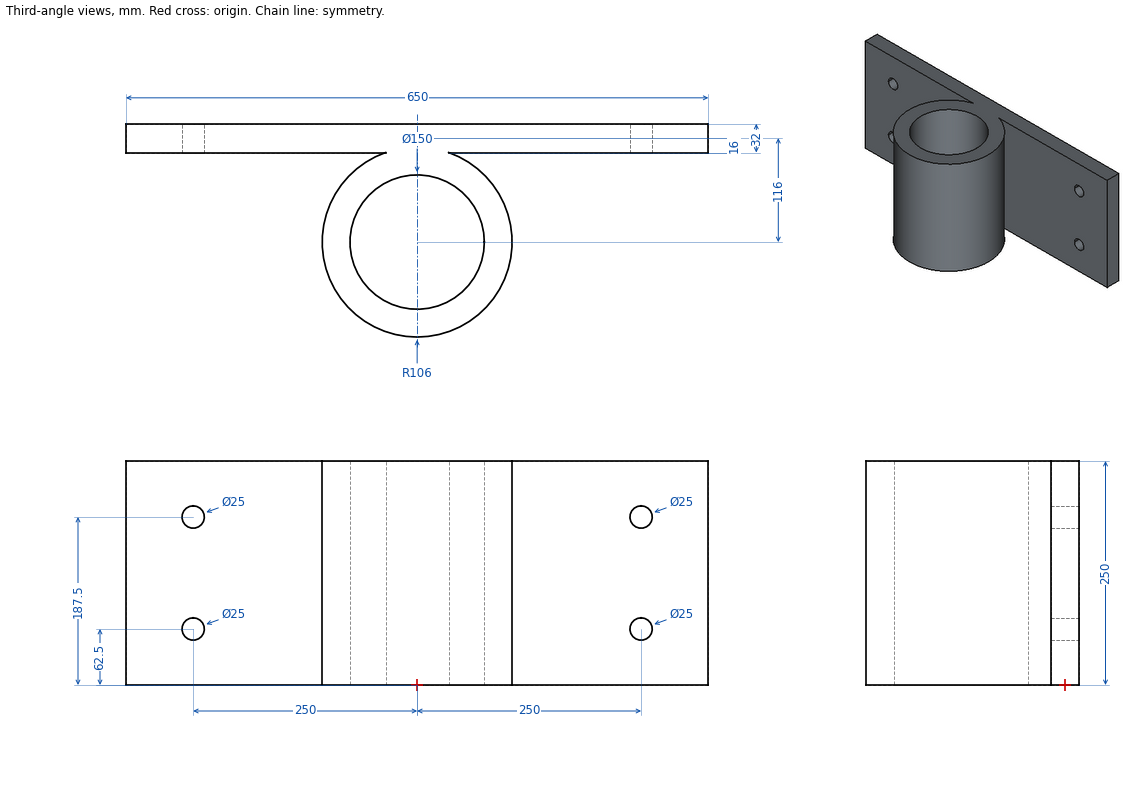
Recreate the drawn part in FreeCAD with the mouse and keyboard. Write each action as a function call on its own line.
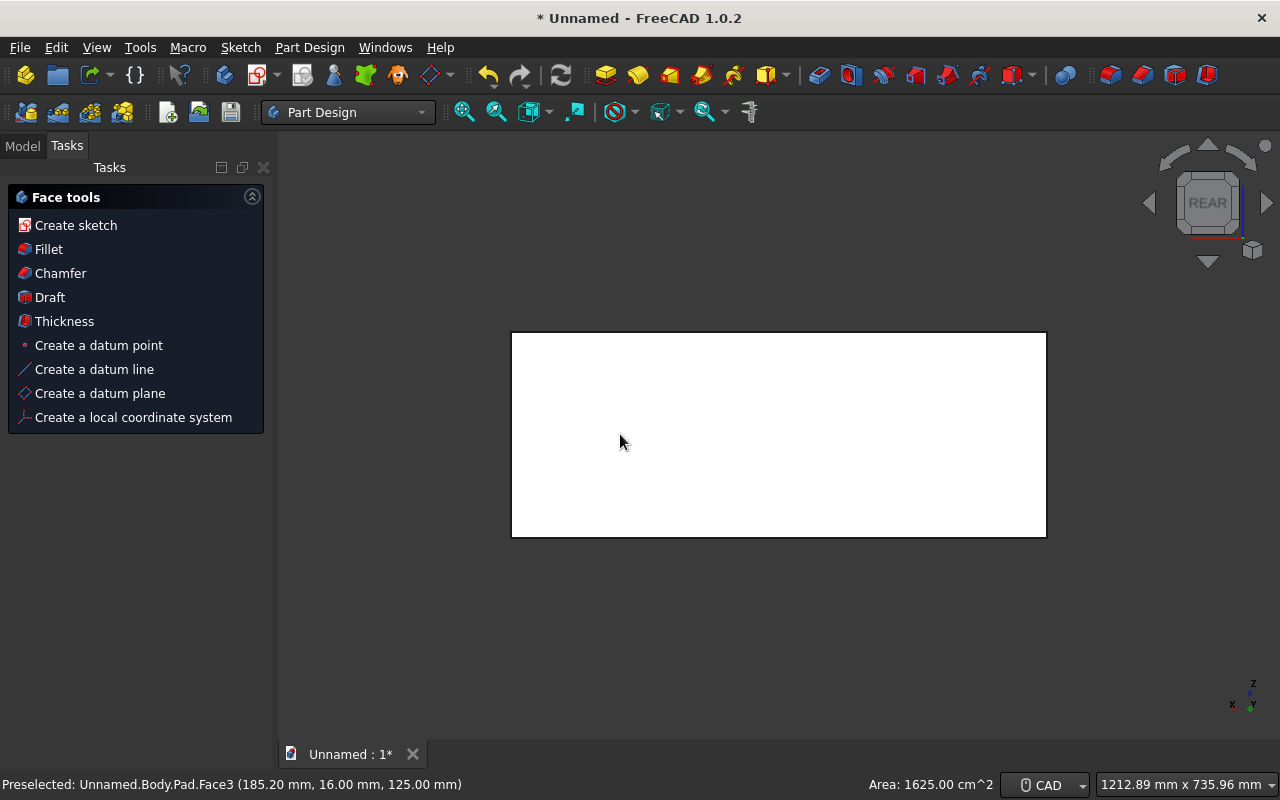
click(258, 76)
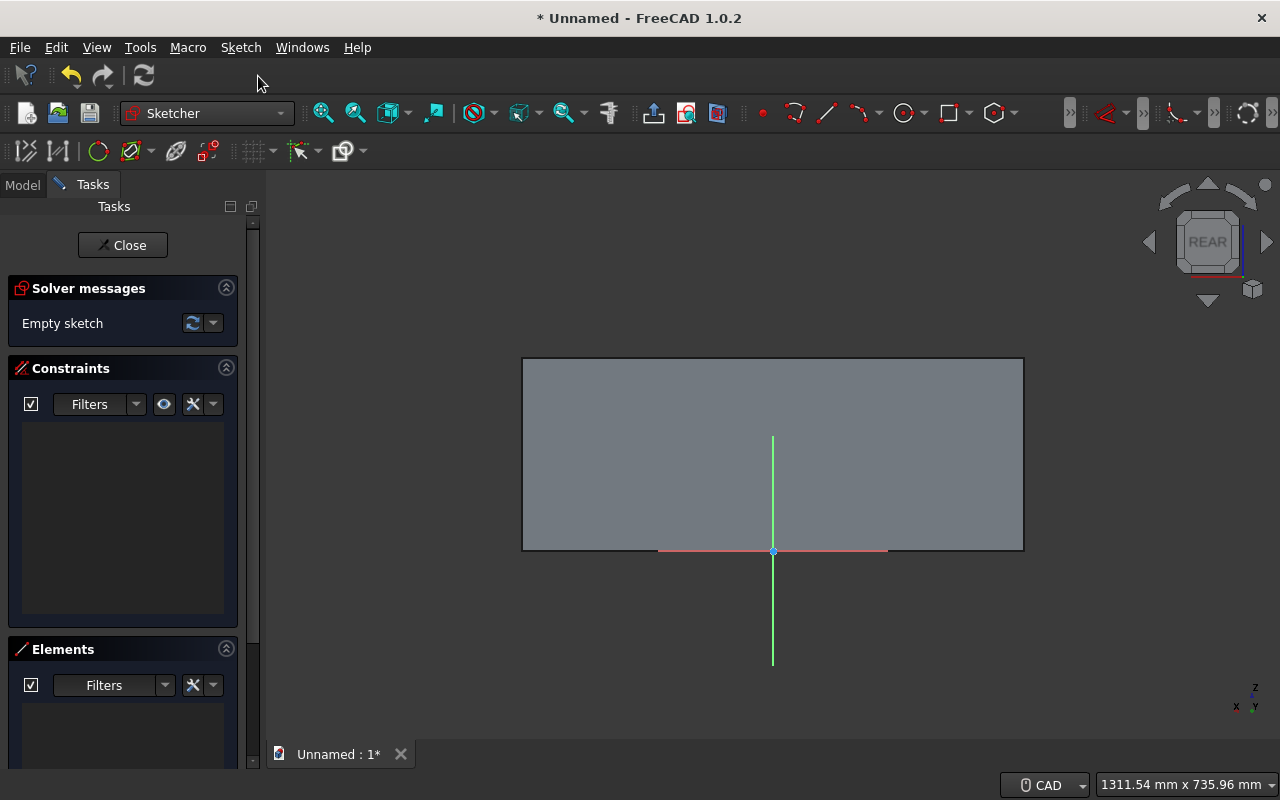
scroll(980, 505, up, 15)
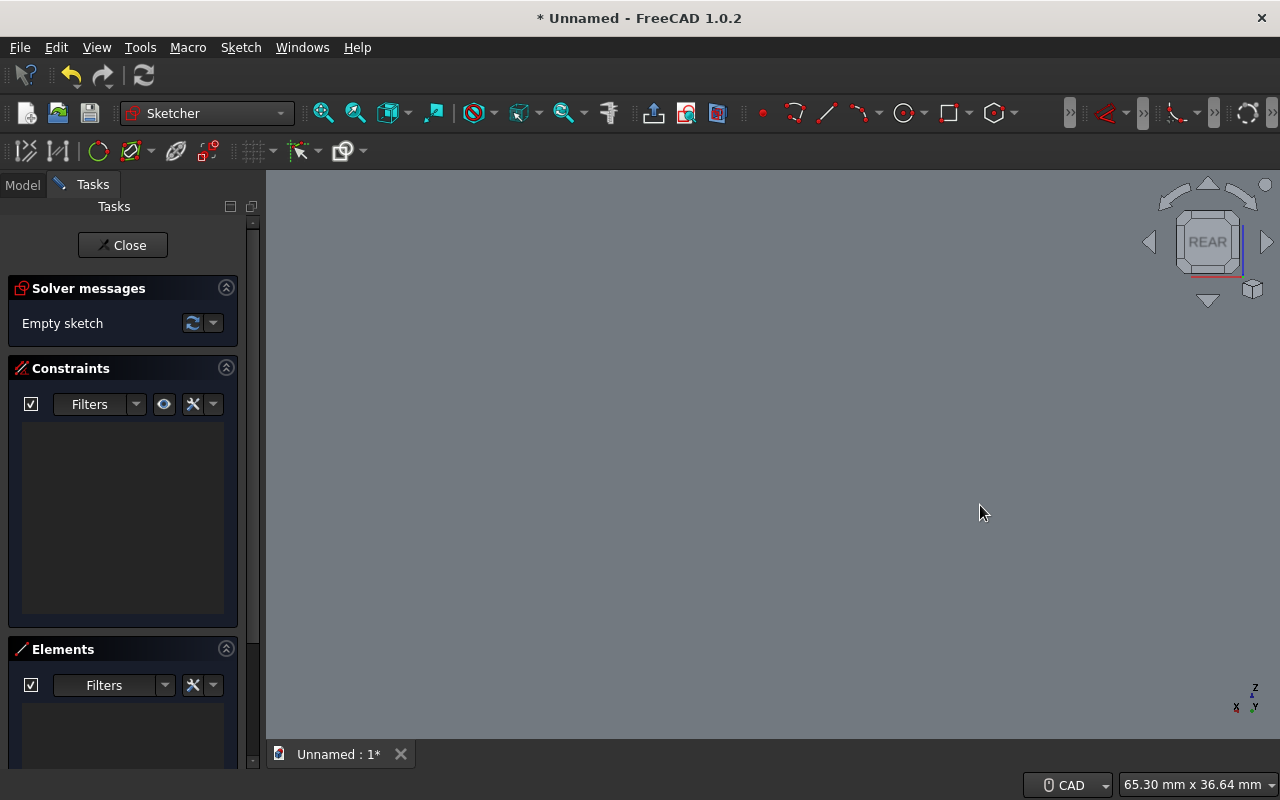
click(904, 114)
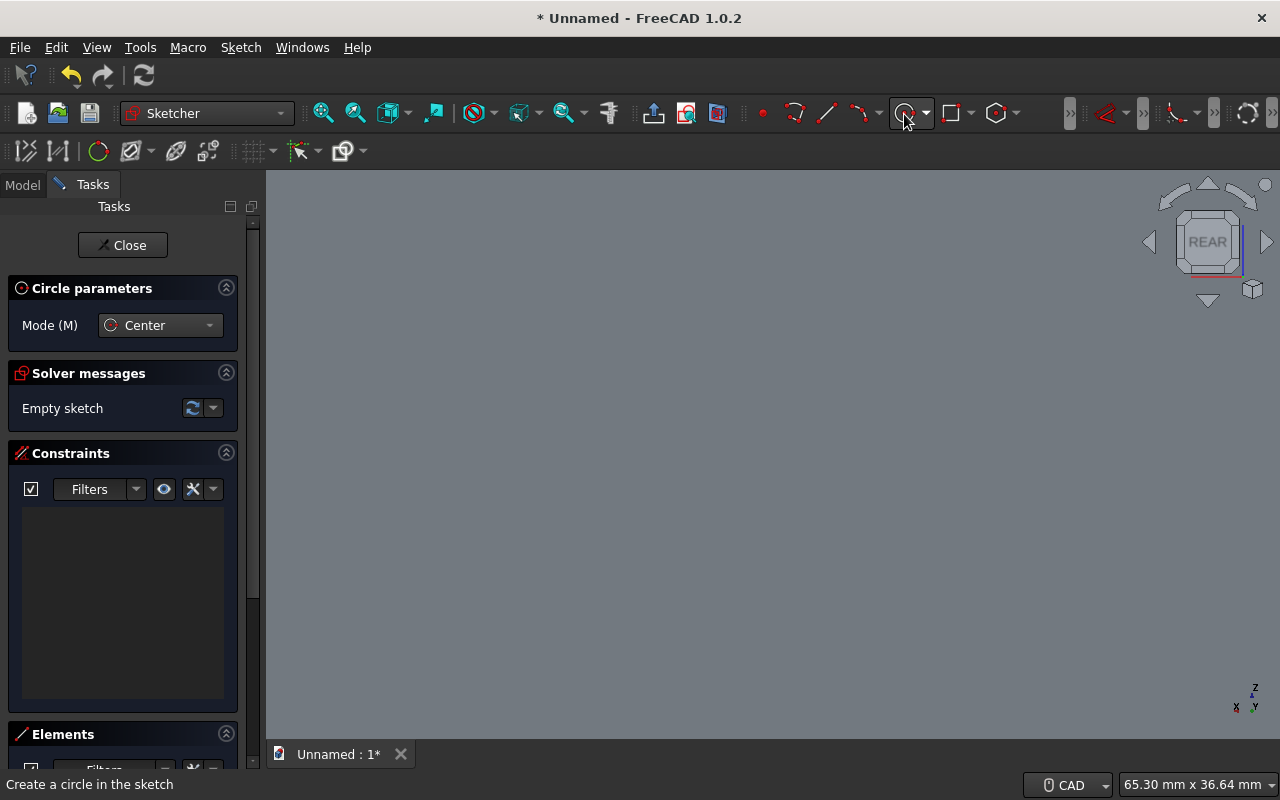
click(691, 450)
click(828, 313)
key(Escape)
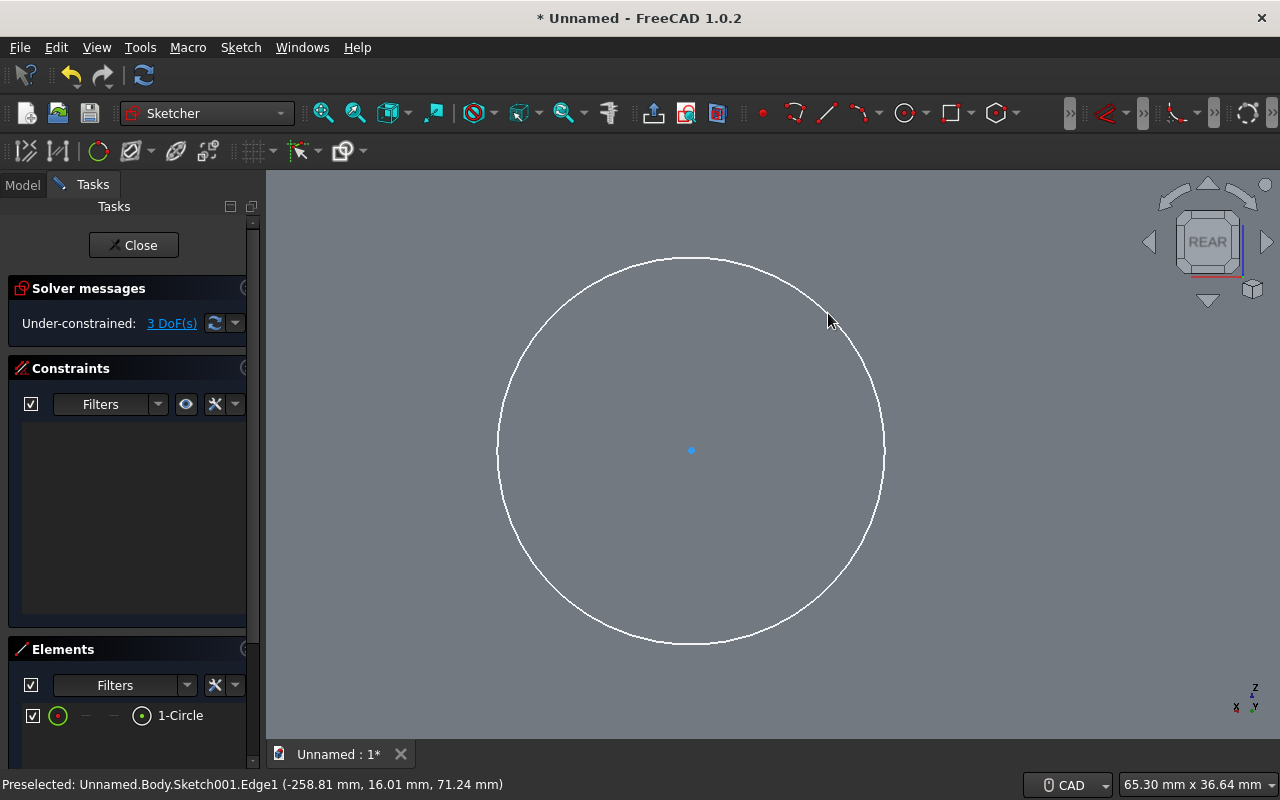
click(1106, 114)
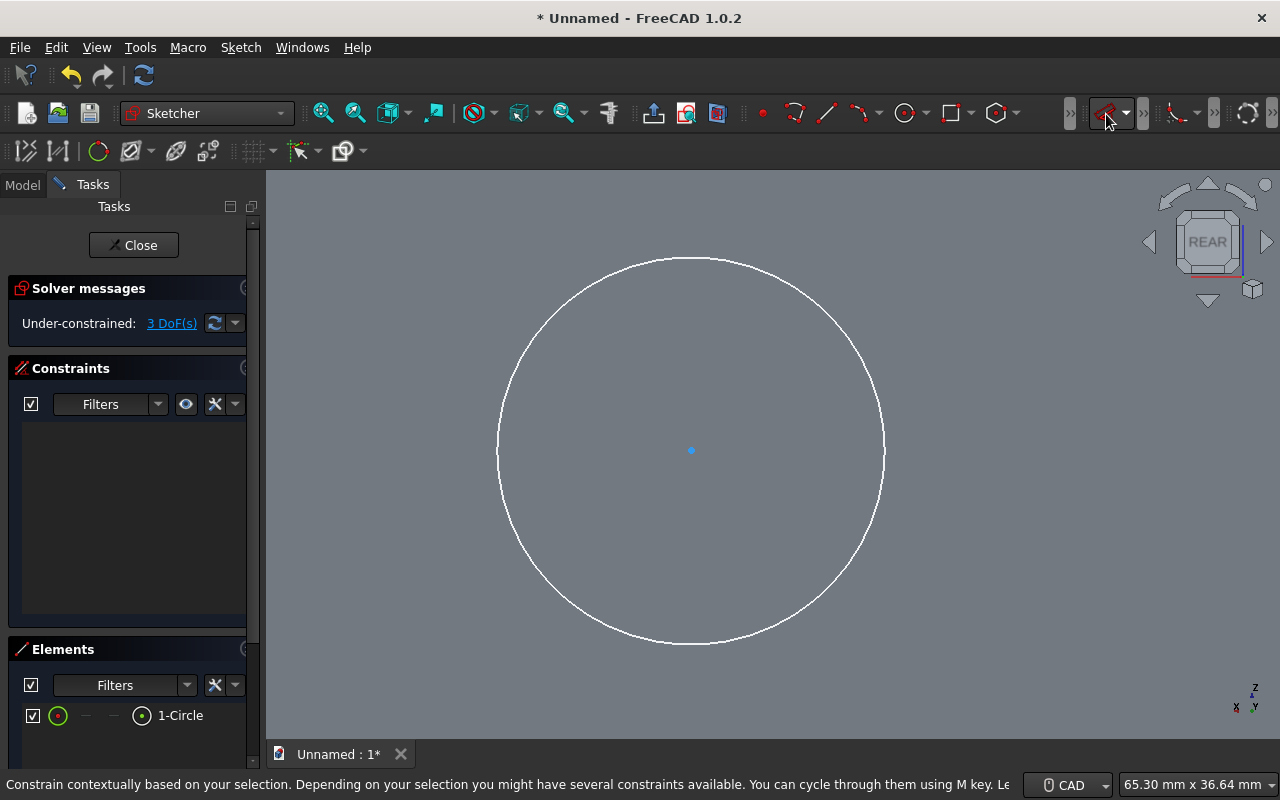
click(828, 314)
click(851, 291)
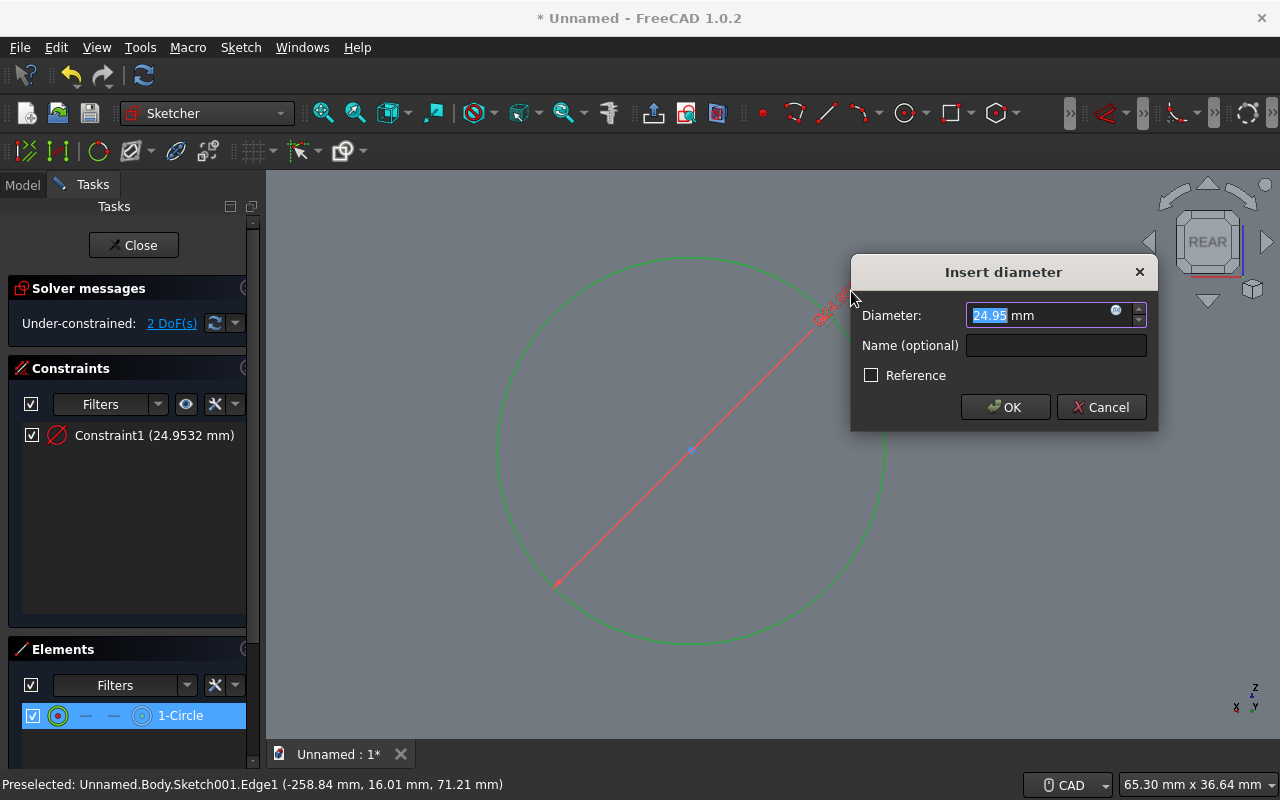
text(25)
key(Return)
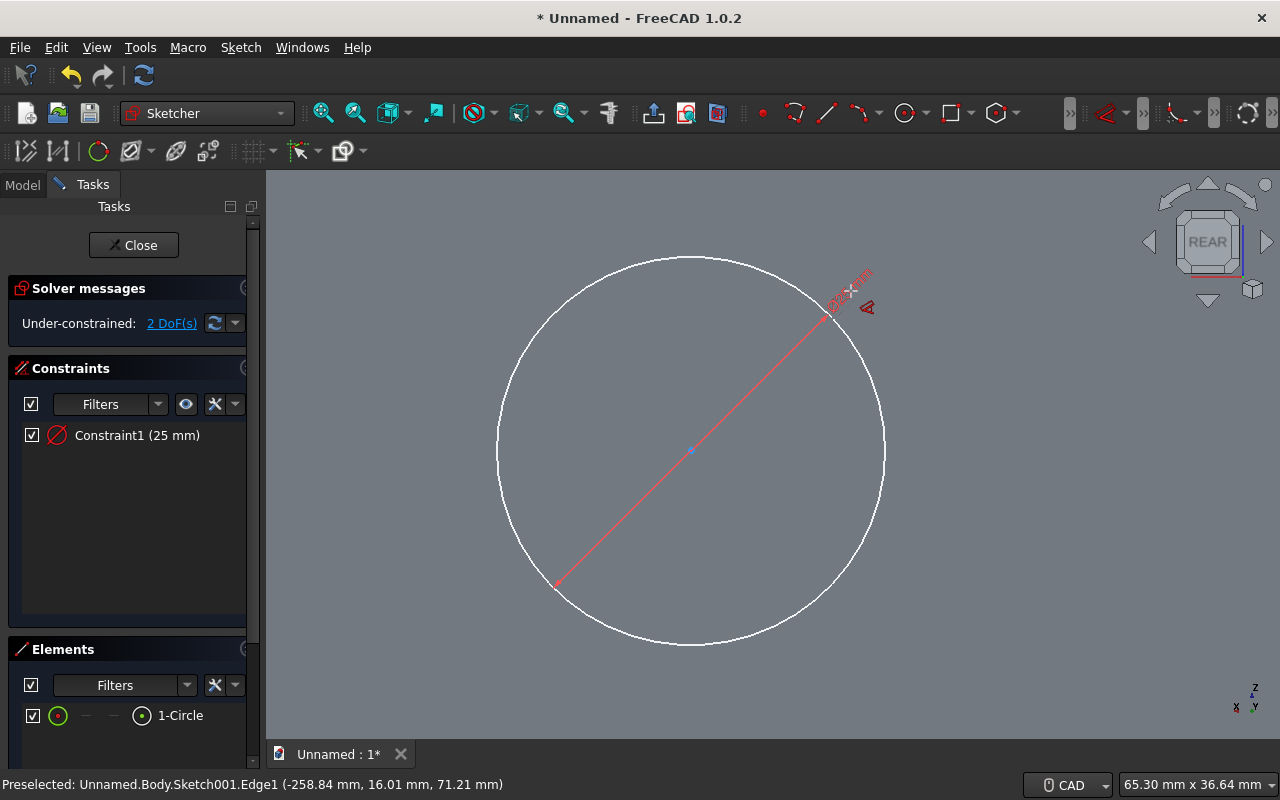
click(691, 451)
click(401, 417)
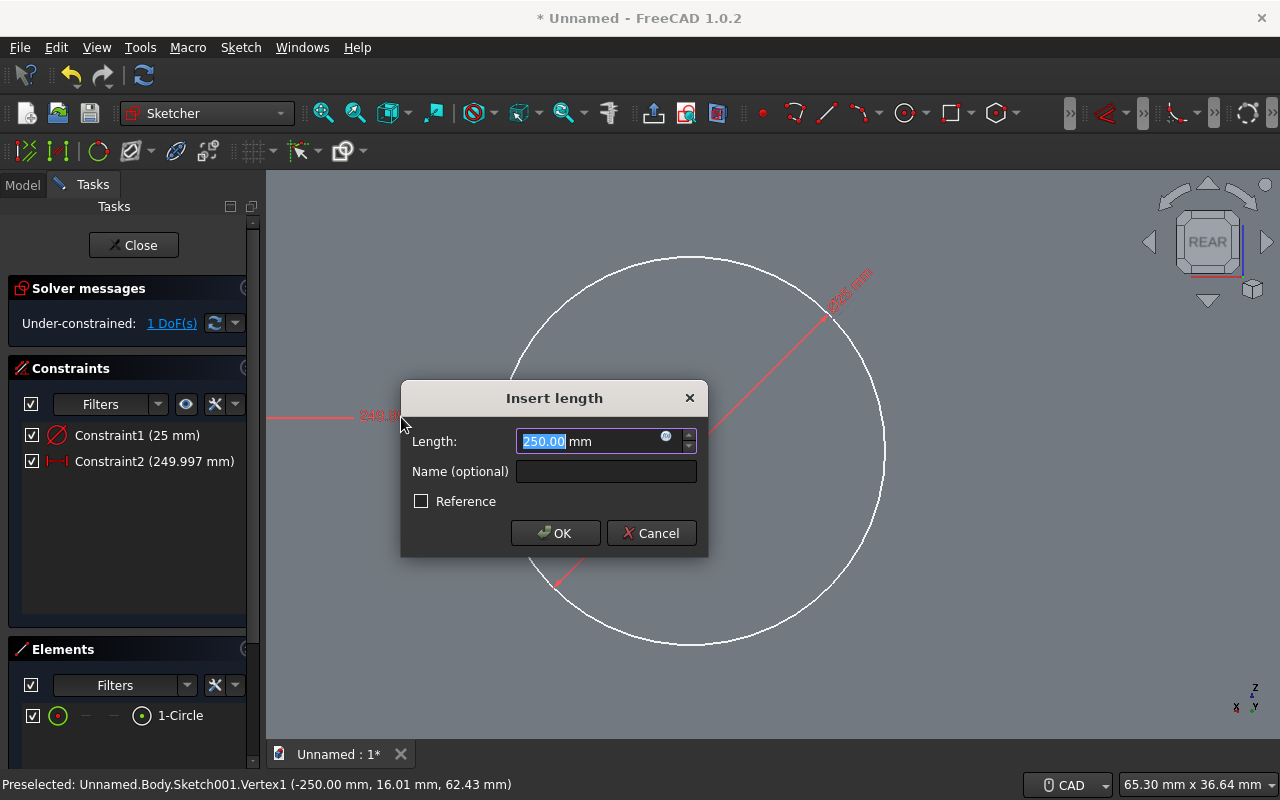
text(250)
key(Return)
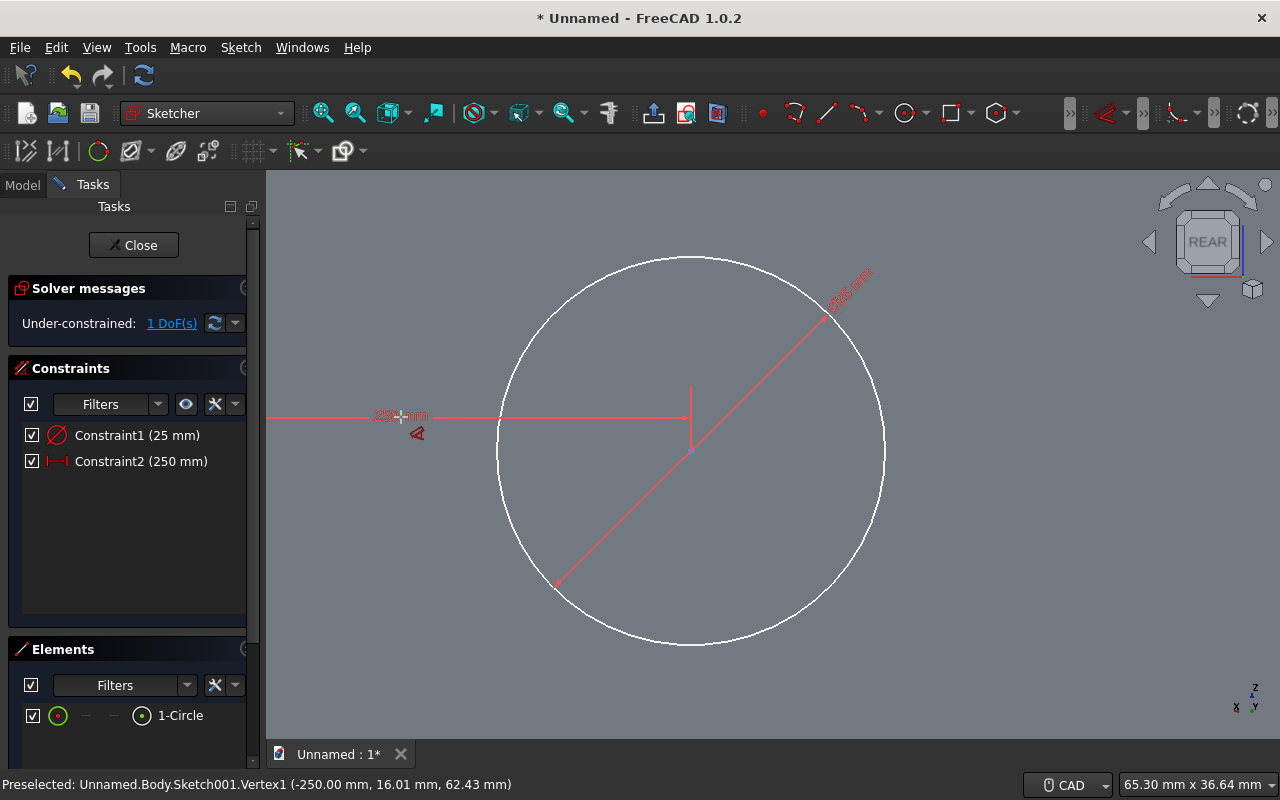
click(691, 451)
click(725, 581)